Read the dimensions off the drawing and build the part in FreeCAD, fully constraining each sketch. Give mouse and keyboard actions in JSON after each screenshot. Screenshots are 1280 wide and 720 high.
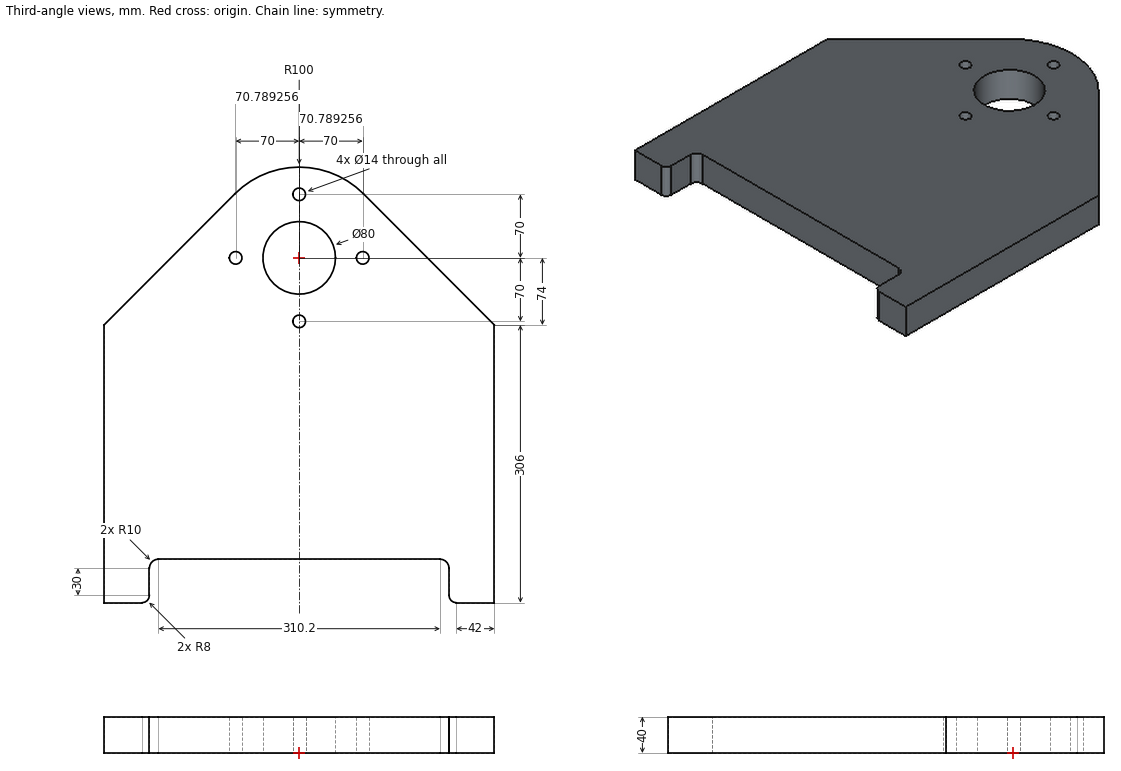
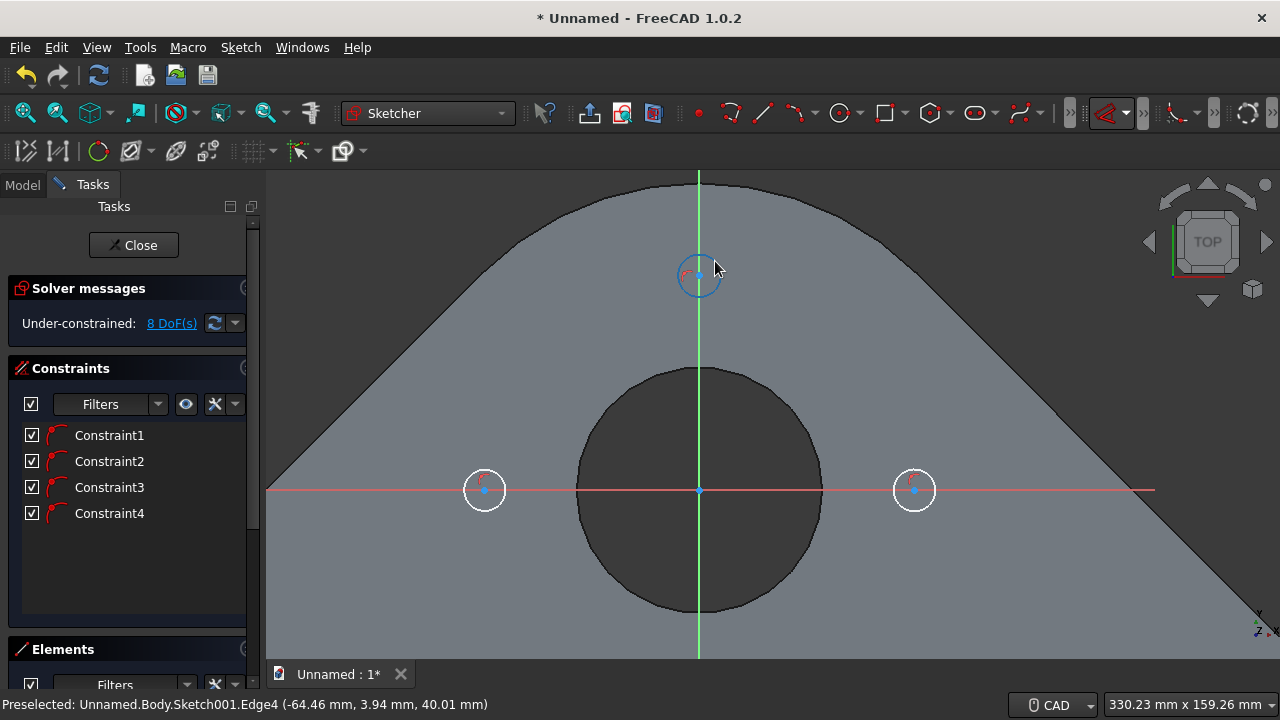
{"action": "left_click", "coordinate": [714, 261]}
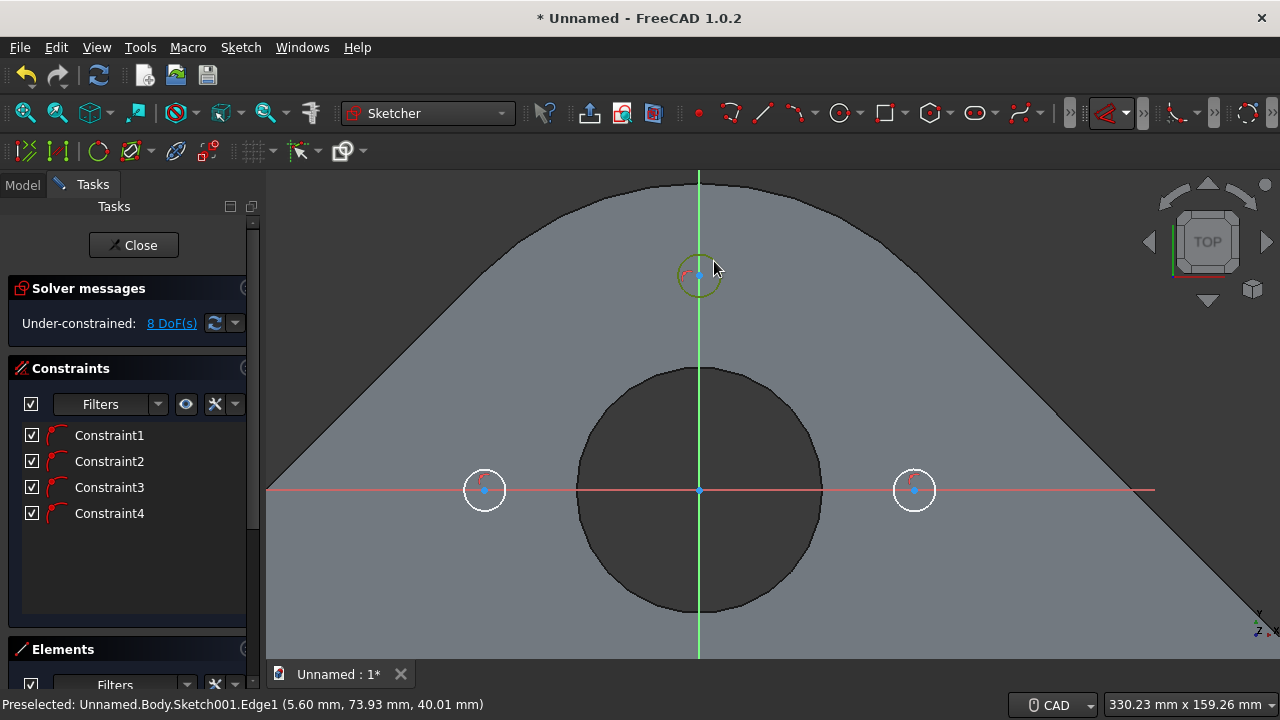
{"action": "left_click", "coordinate": [929, 476]}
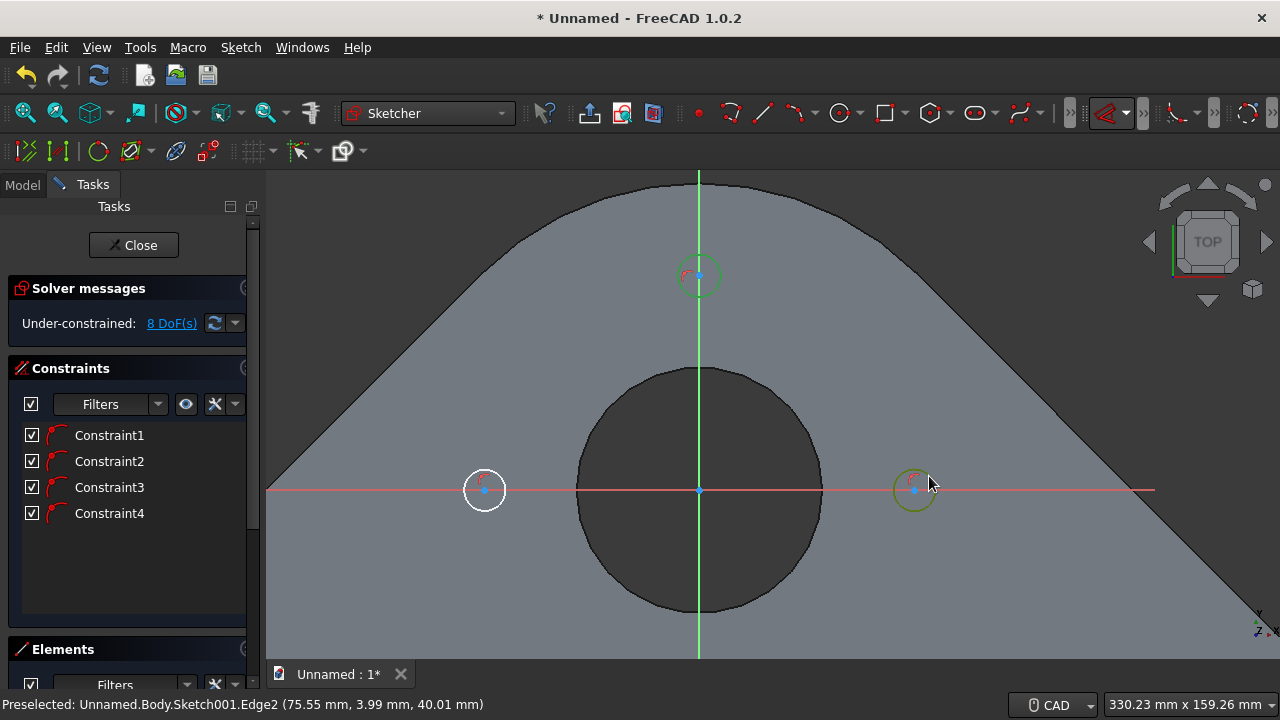
{"action": "scroll", "coordinate": [715, 260], "scroll_direction": "down", "scroll_amount": 2}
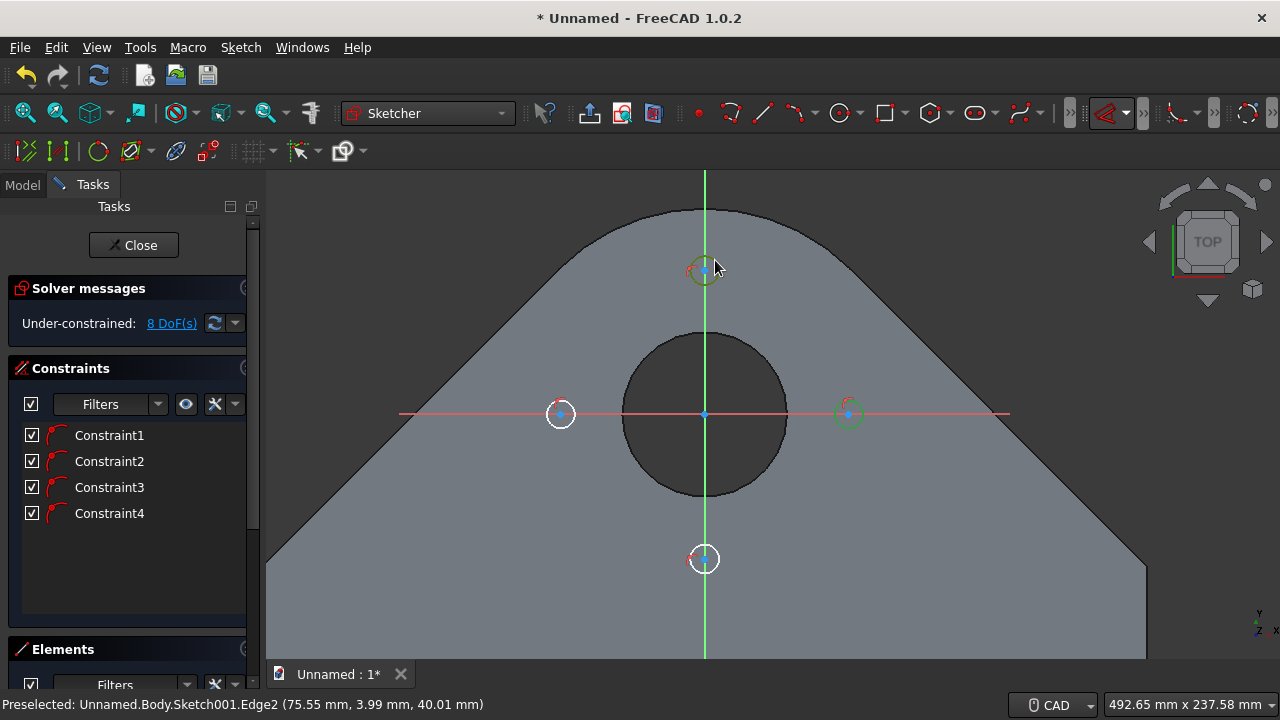
{"action": "scroll", "coordinate": [715, 549], "scroll_direction": "up", "scroll_amount": 2}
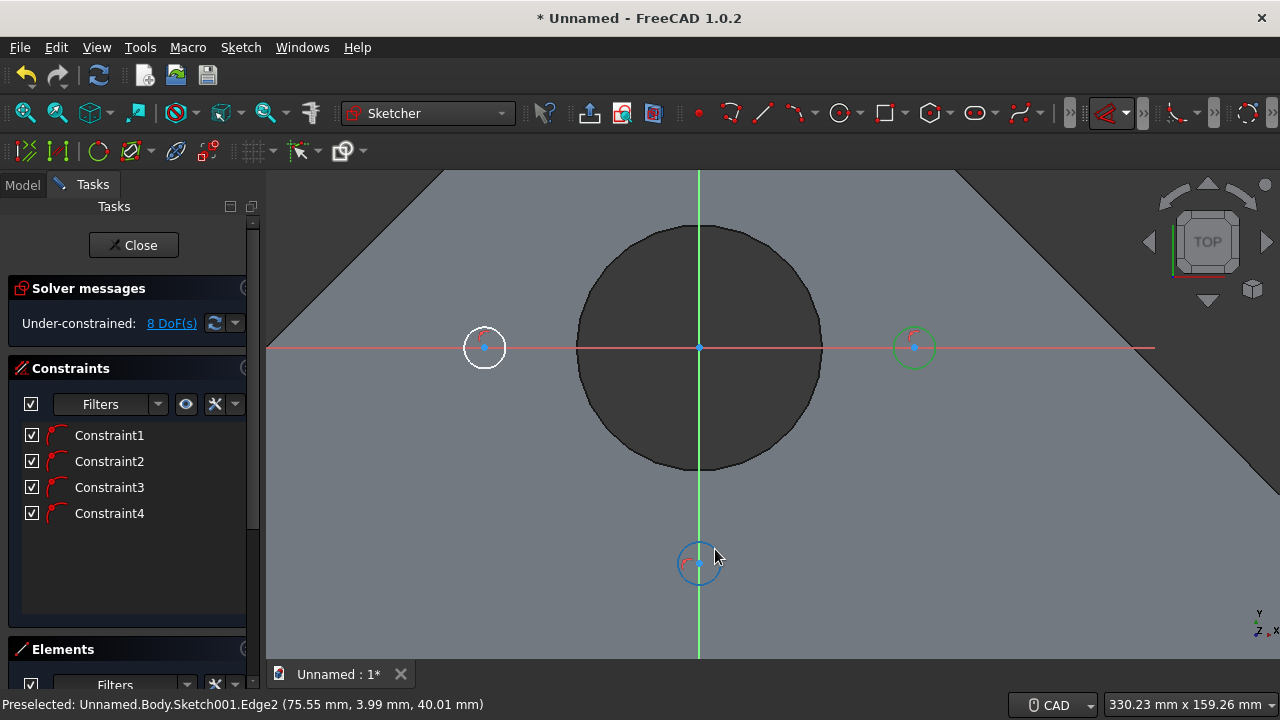
{"action": "left_click", "coordinate": [714, 548]}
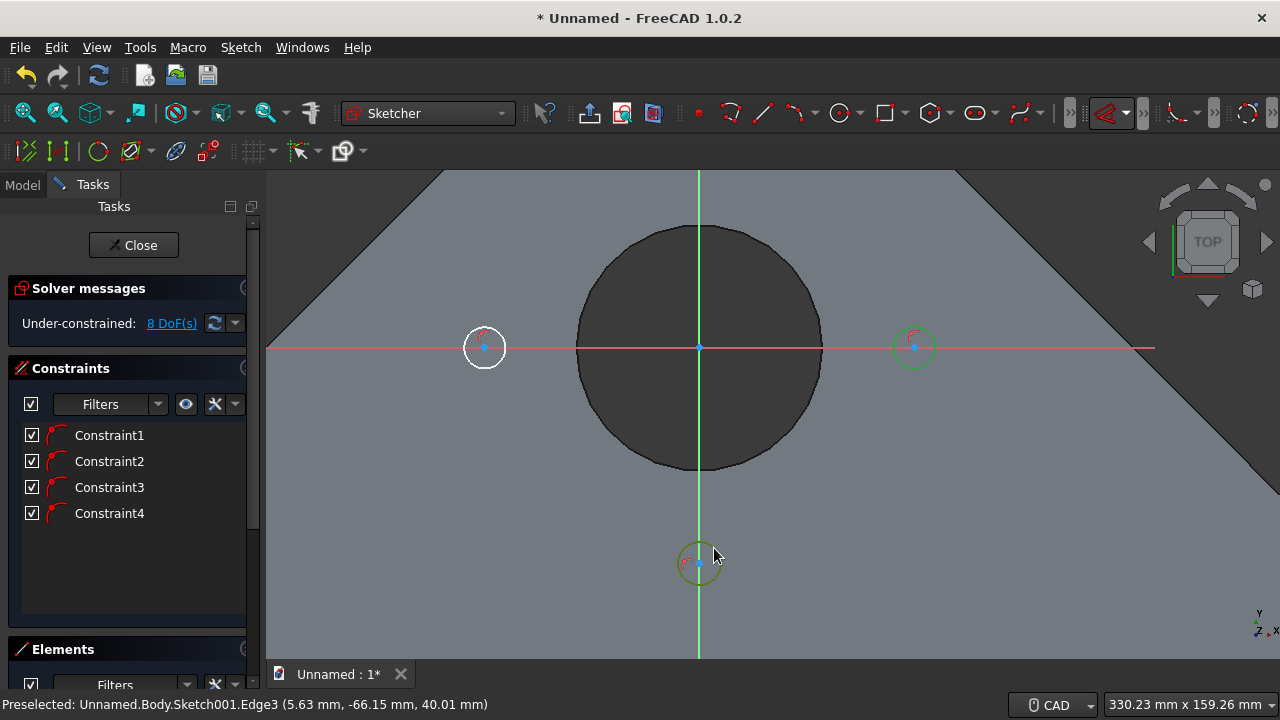
{"action": "left_click", "coordinate": [499, 333]}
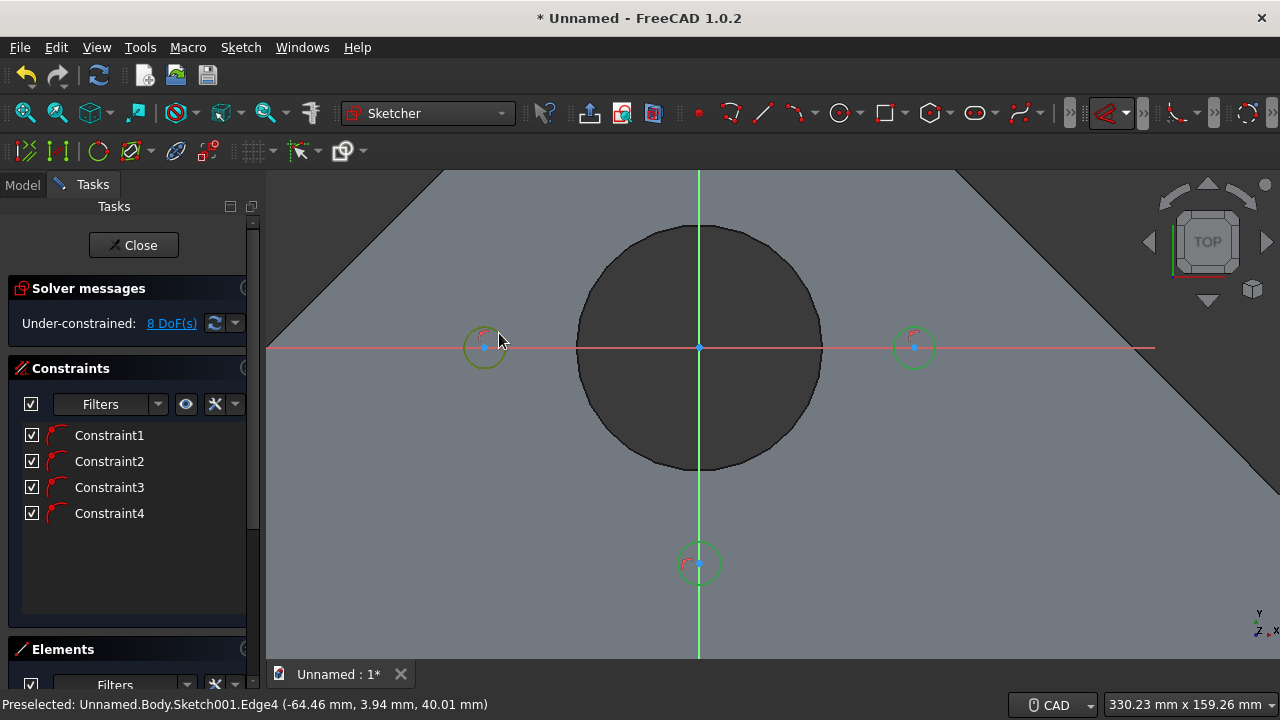
{"action": "key", "text": "e"}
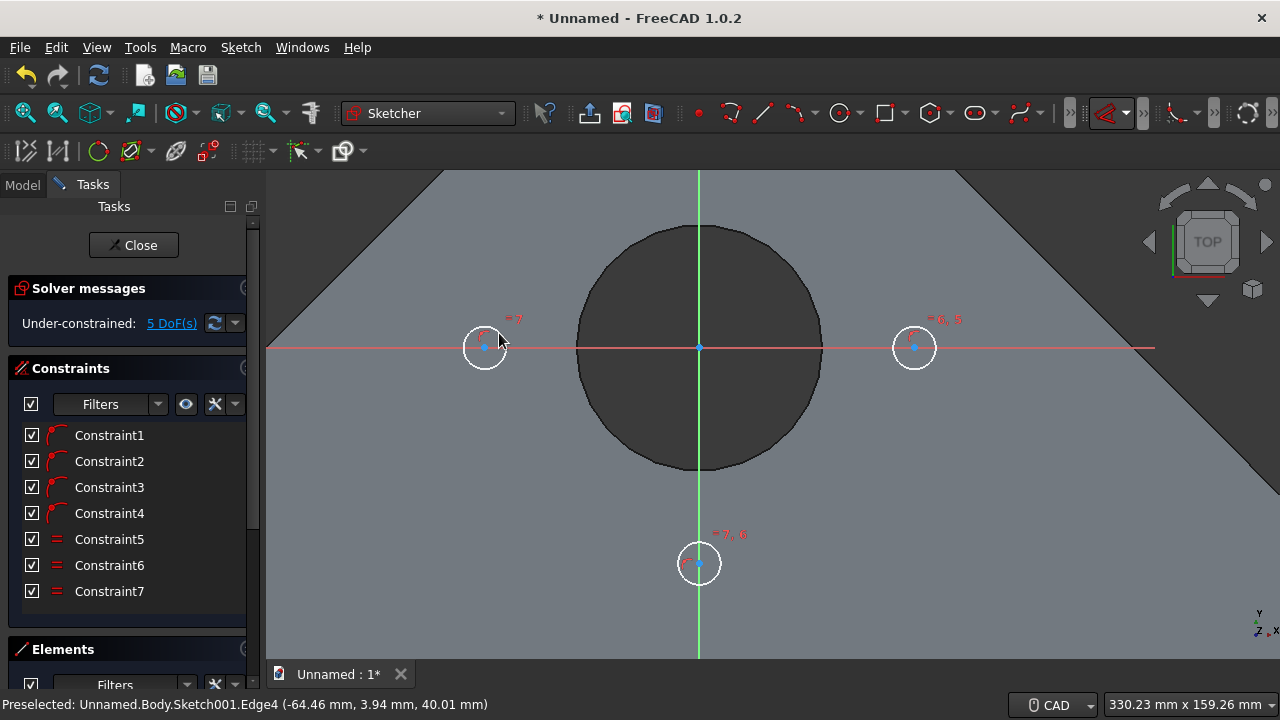
{"action": "key", "text": "d"}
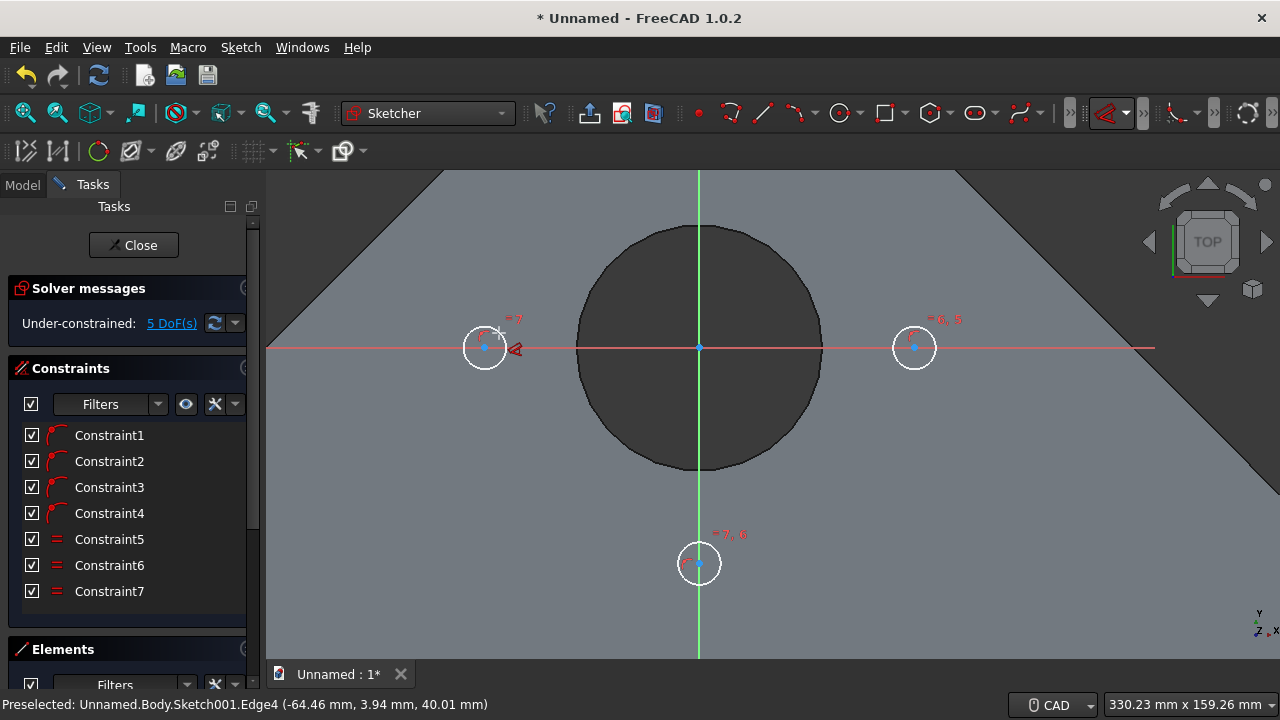
{"action": "scroll", "coordinate": [715, 550], "scroll_direction": "down", "scroll_amount": 2}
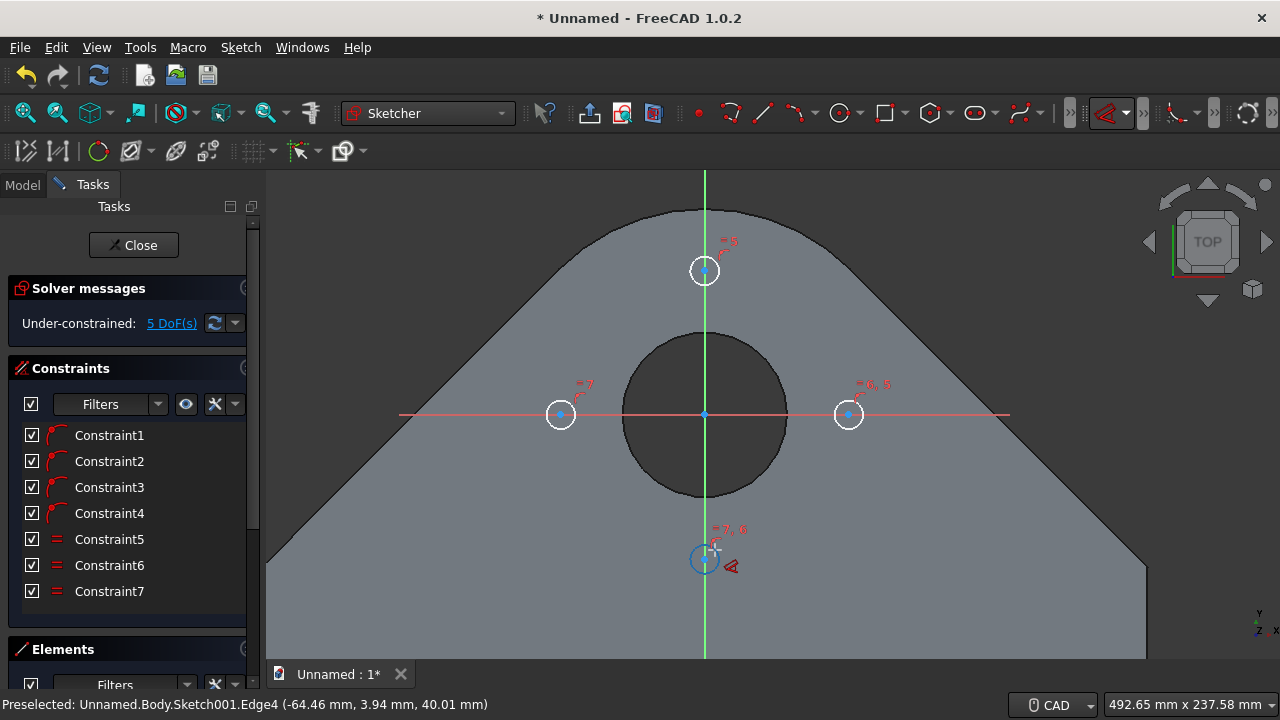
{"action": "scroll", "coordinate": [715, 261], "scroll_direction": "up", "scroll_amount": 2}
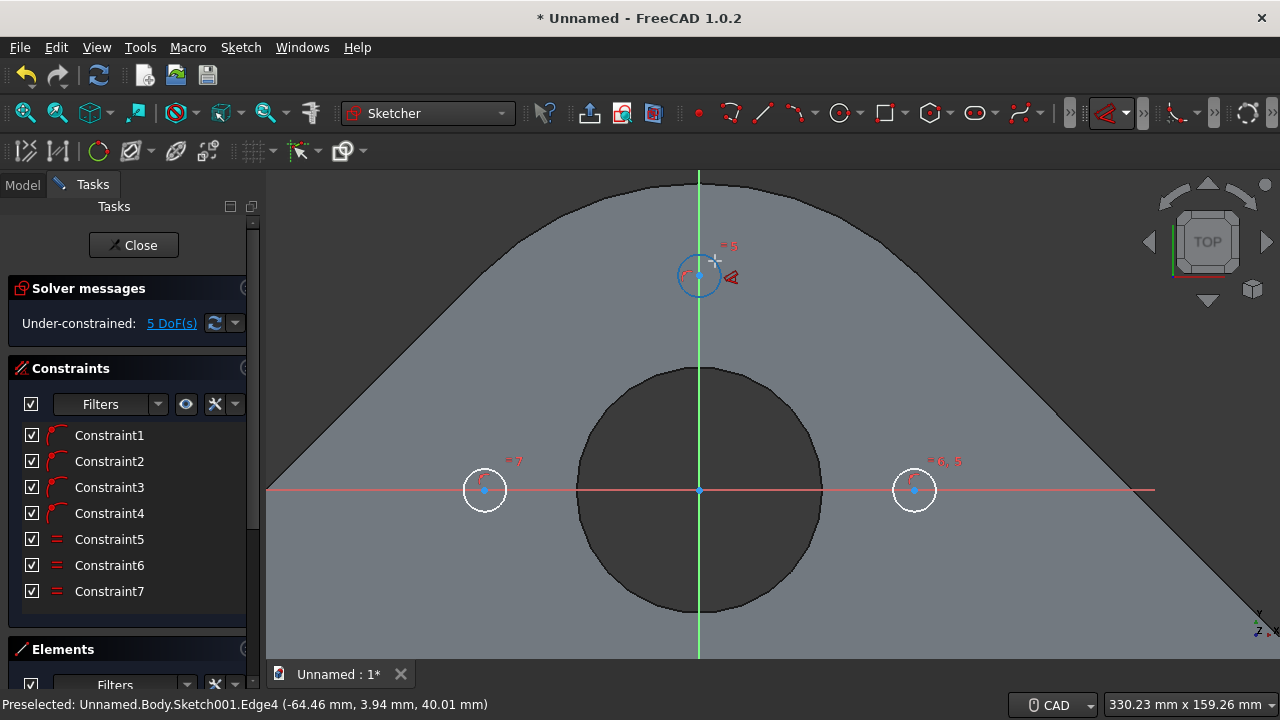
{"action": "left_click", "coordinate": [714, 261]}
{"action": "left_click", "coordinate": [736, 238]}